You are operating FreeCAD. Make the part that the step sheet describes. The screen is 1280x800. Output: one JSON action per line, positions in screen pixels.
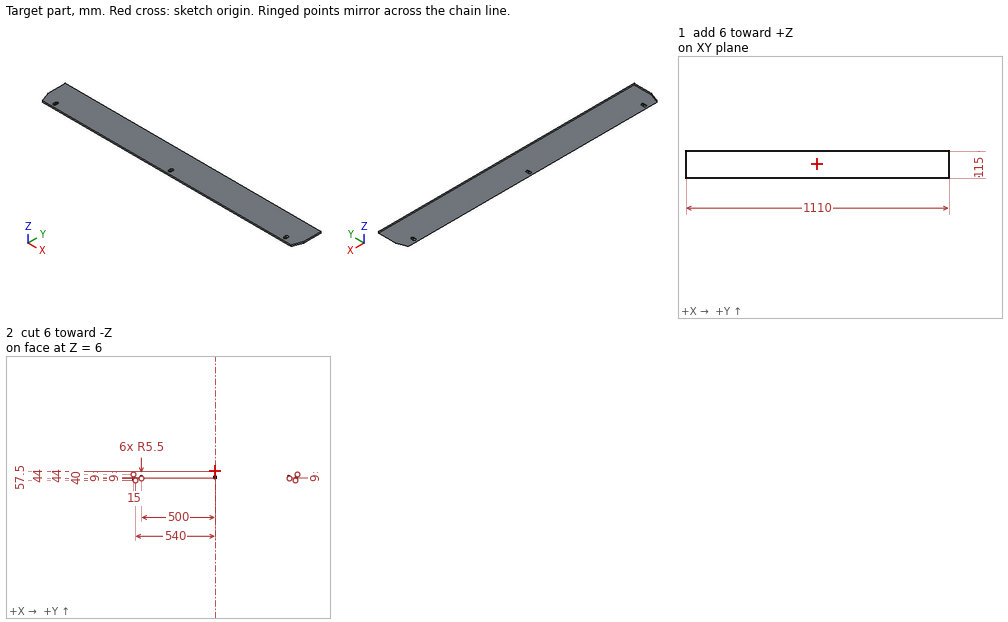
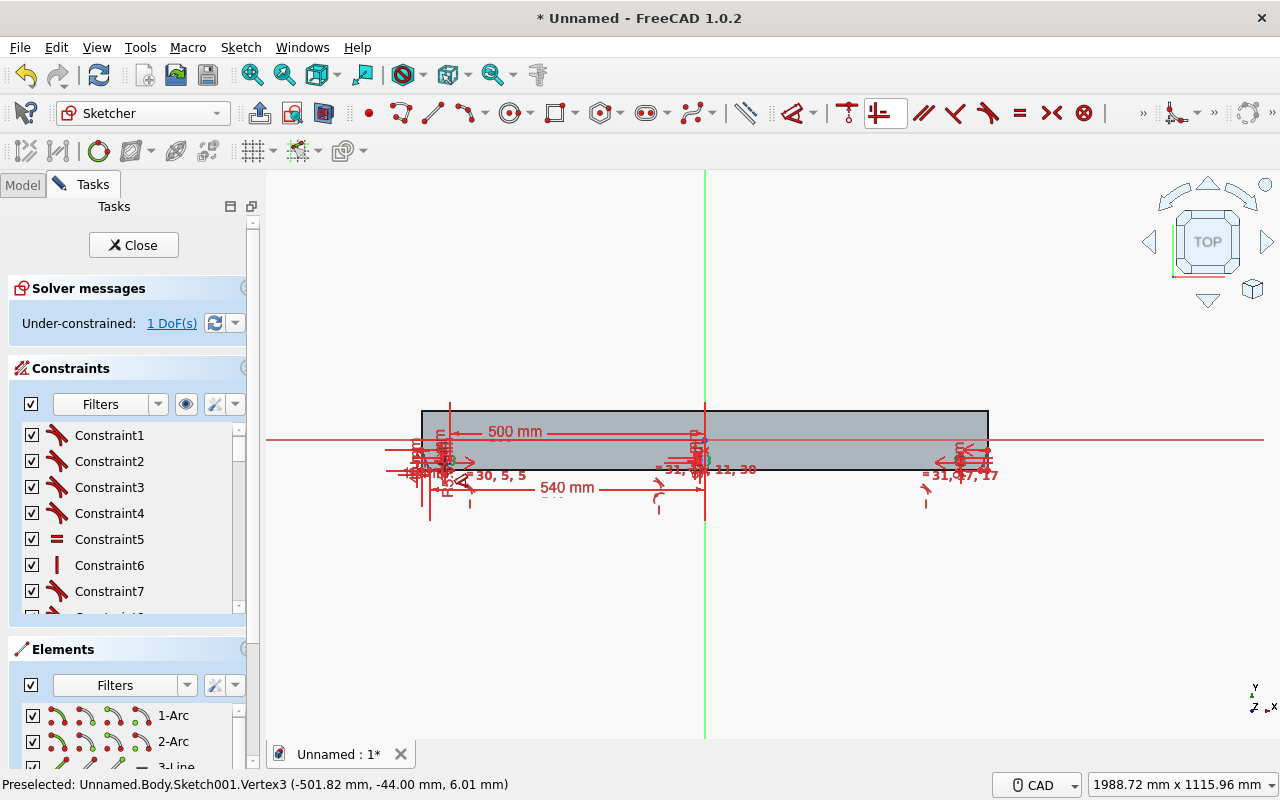
{"action": "scroll", "coordinate": [430, 471], "scroll_direction": "up", "scroll_amount": 3}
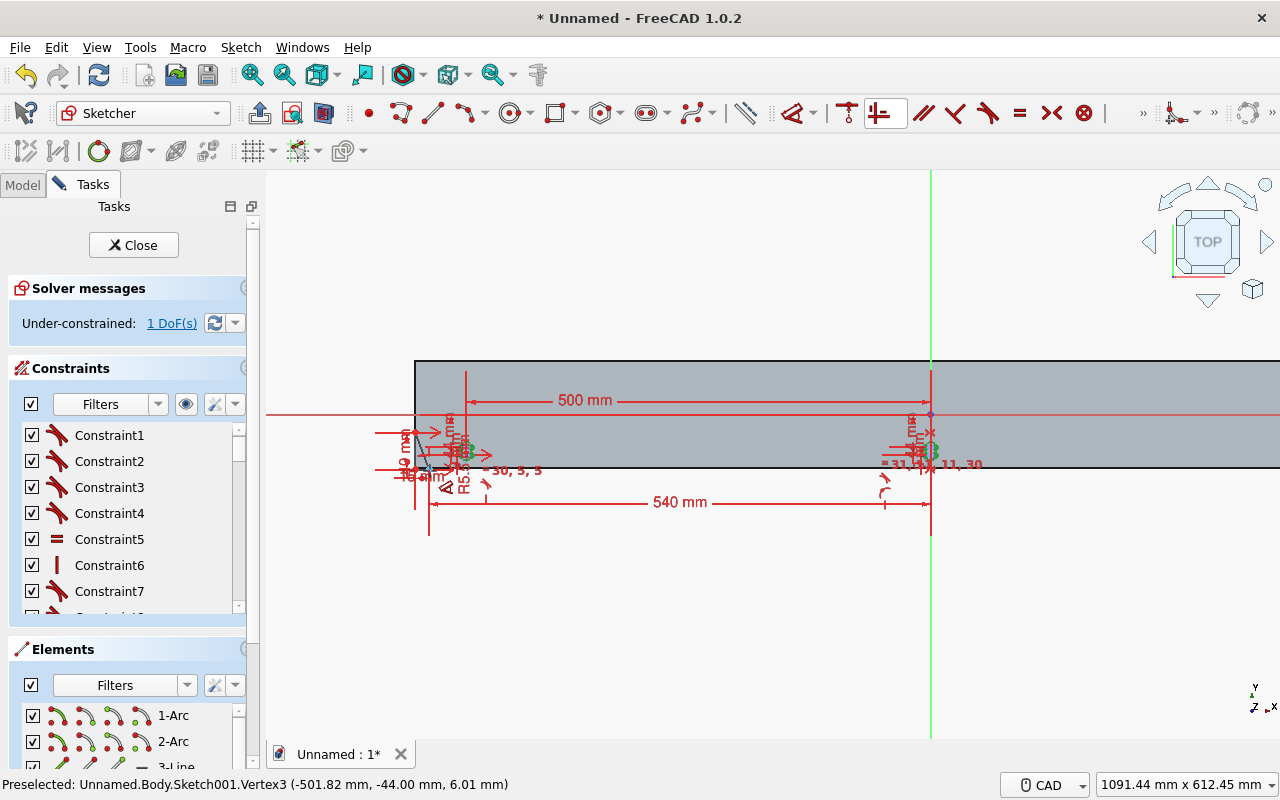
{"action": "left_click", "coordinate": [429, 470]}
{"action": "left_click", "coordinate": [371, 429]}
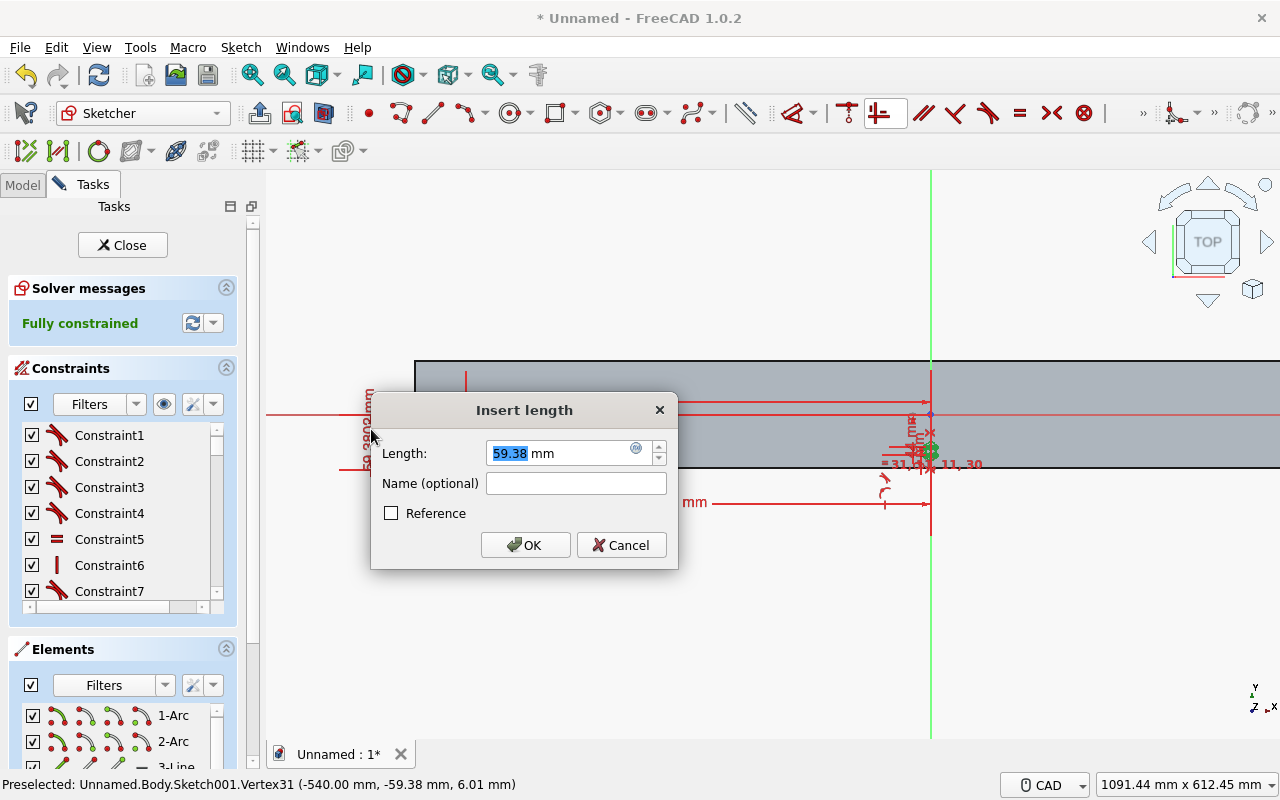
{"action": "type", "text": "57.5"}
{"action": "key", "text": "Return"}
{"action": "key", "text": "Escape"}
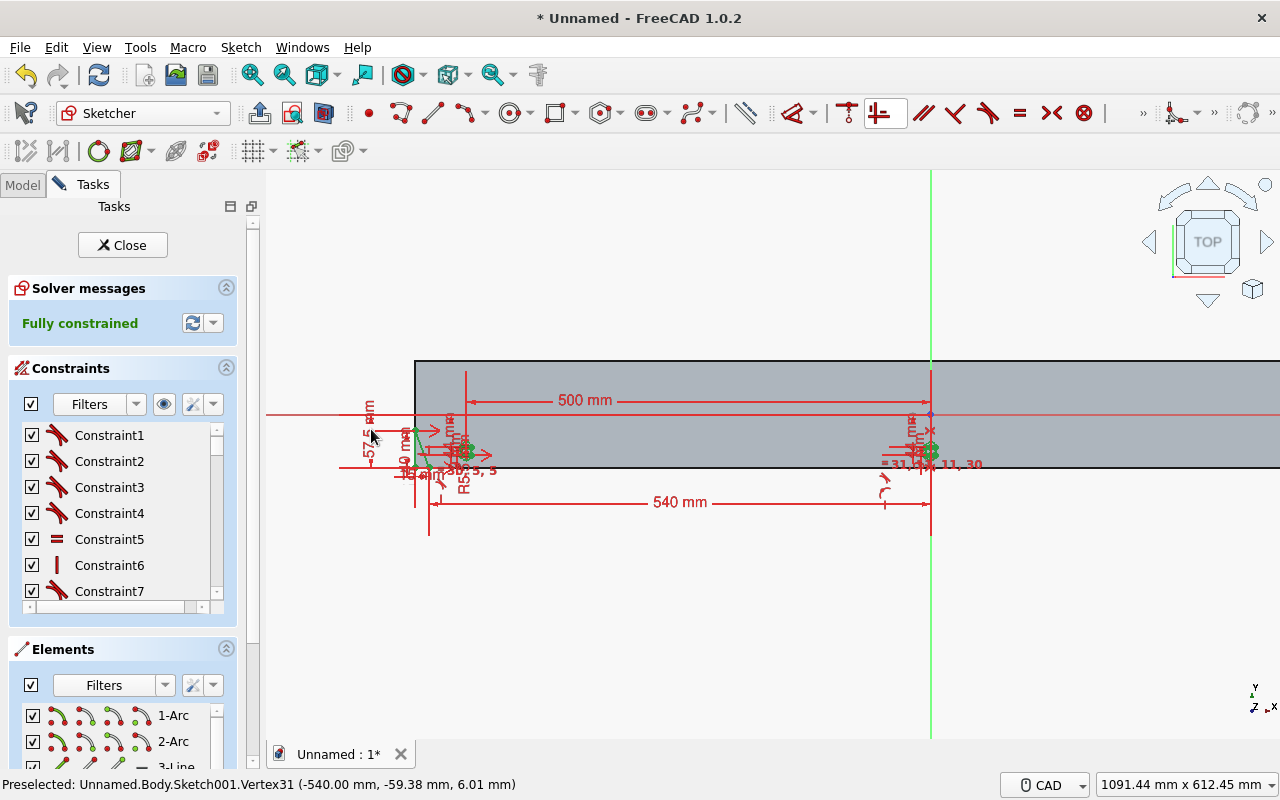
{"action": "left_click", "coordinate": [123, 245]}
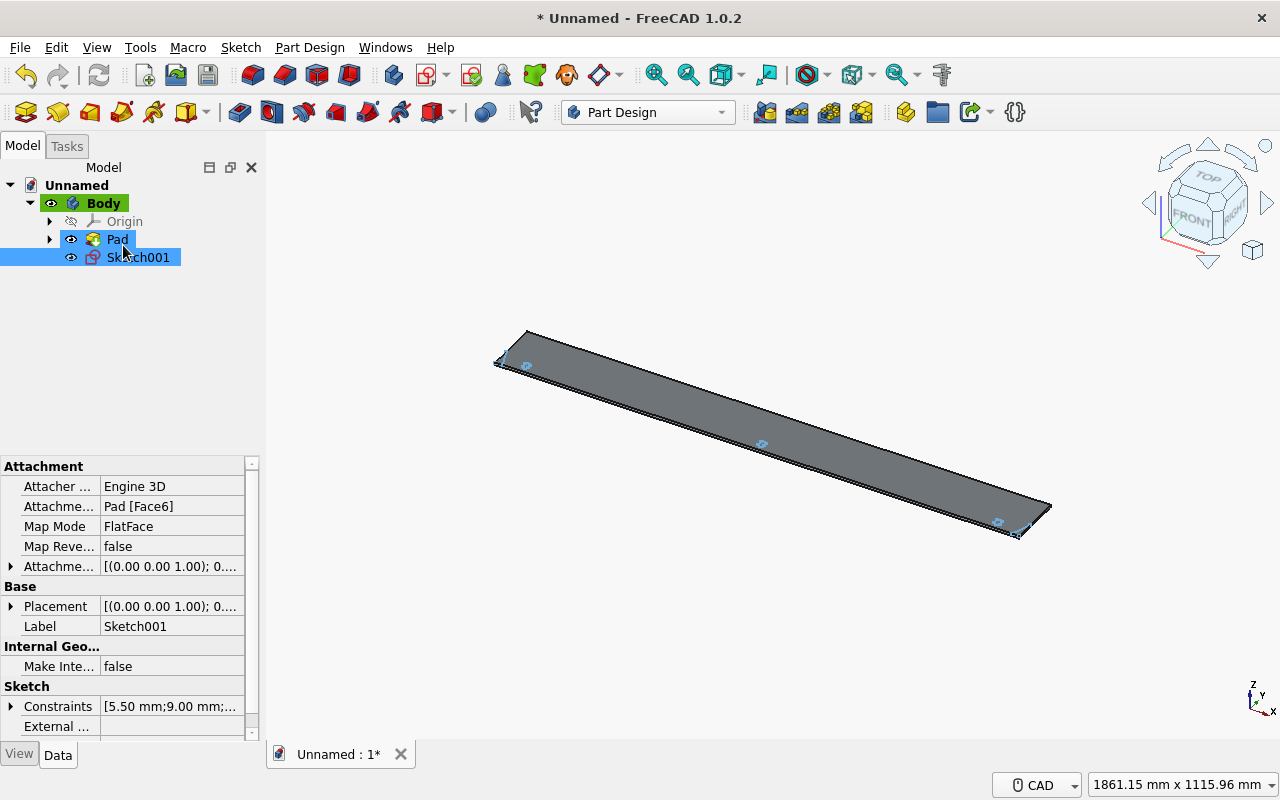
{"action": "left_click", "coordinate": [240, 112]}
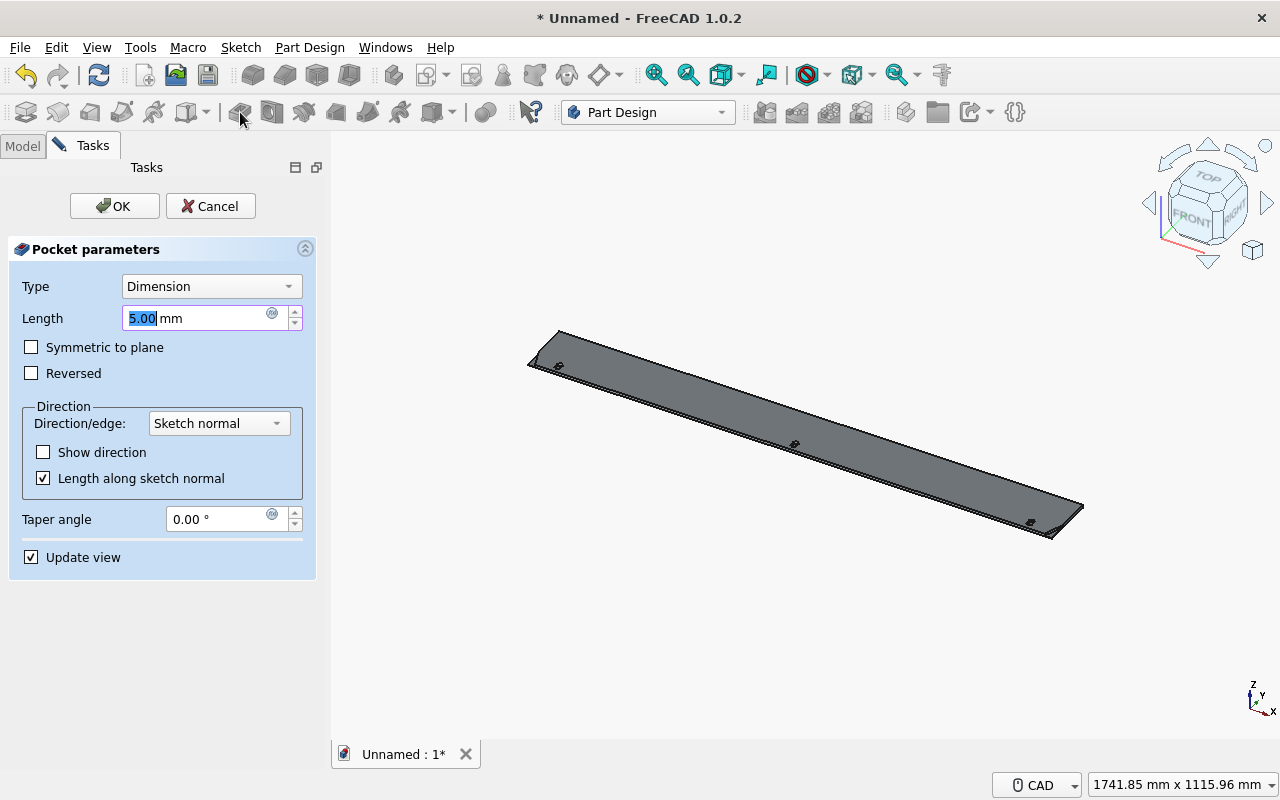
{"action": "type", "text": "6"}
{"action": "key", "text": "Tab"}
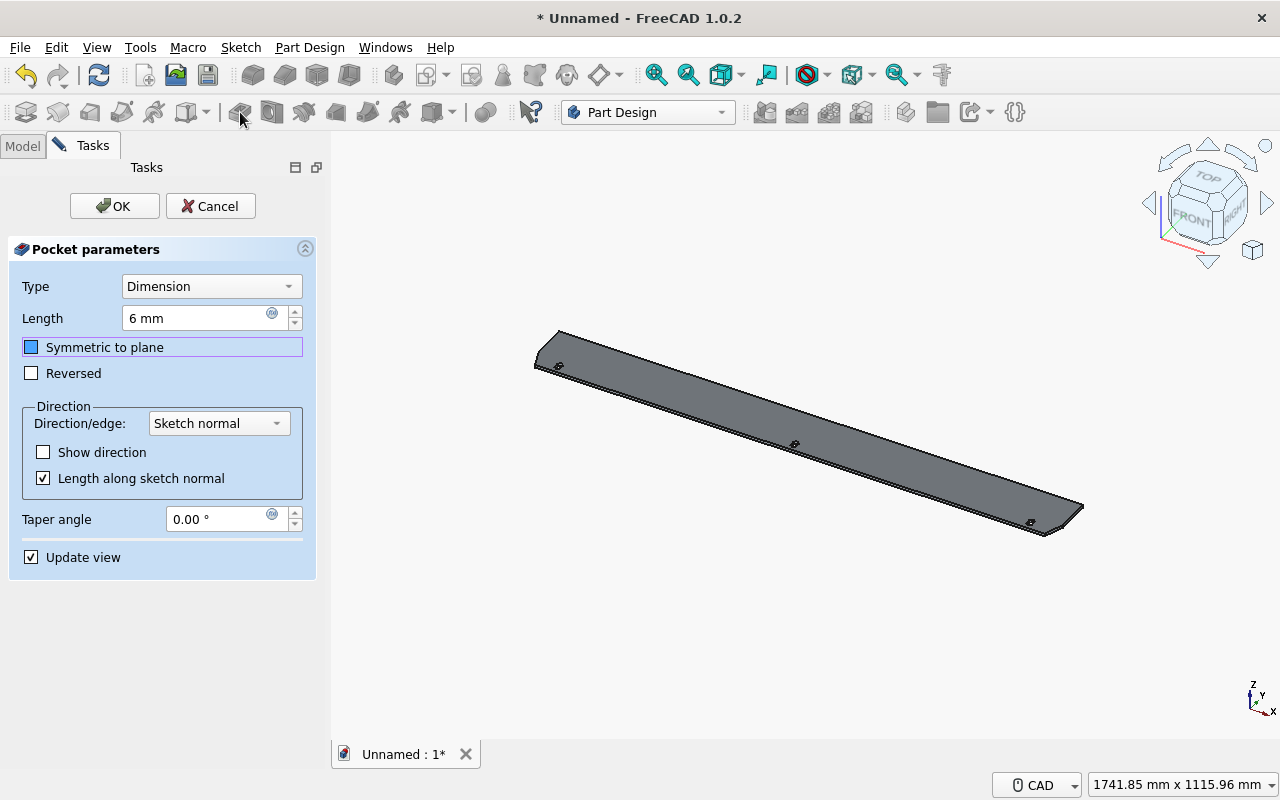
{"action": "left_click", "coordinate": [115, 206]}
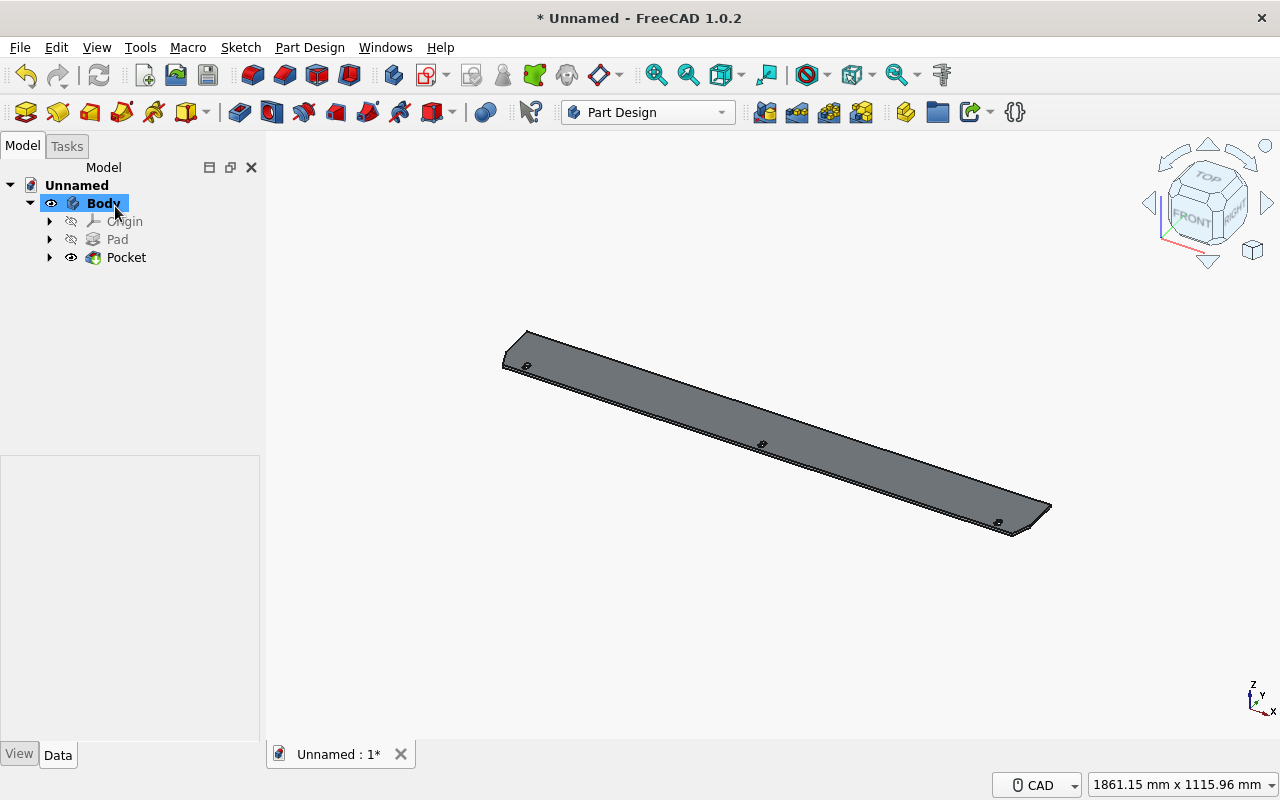
{"action": "key", "text": "0"}